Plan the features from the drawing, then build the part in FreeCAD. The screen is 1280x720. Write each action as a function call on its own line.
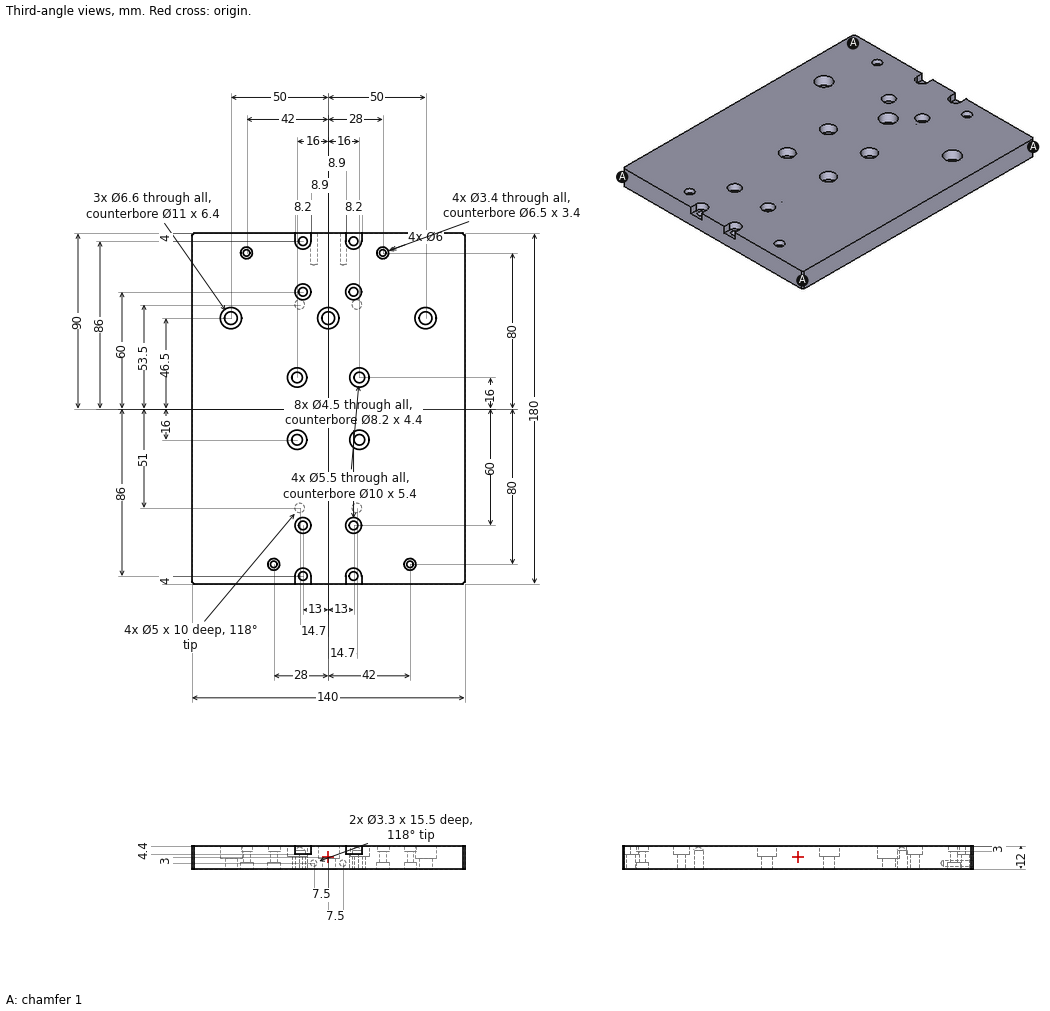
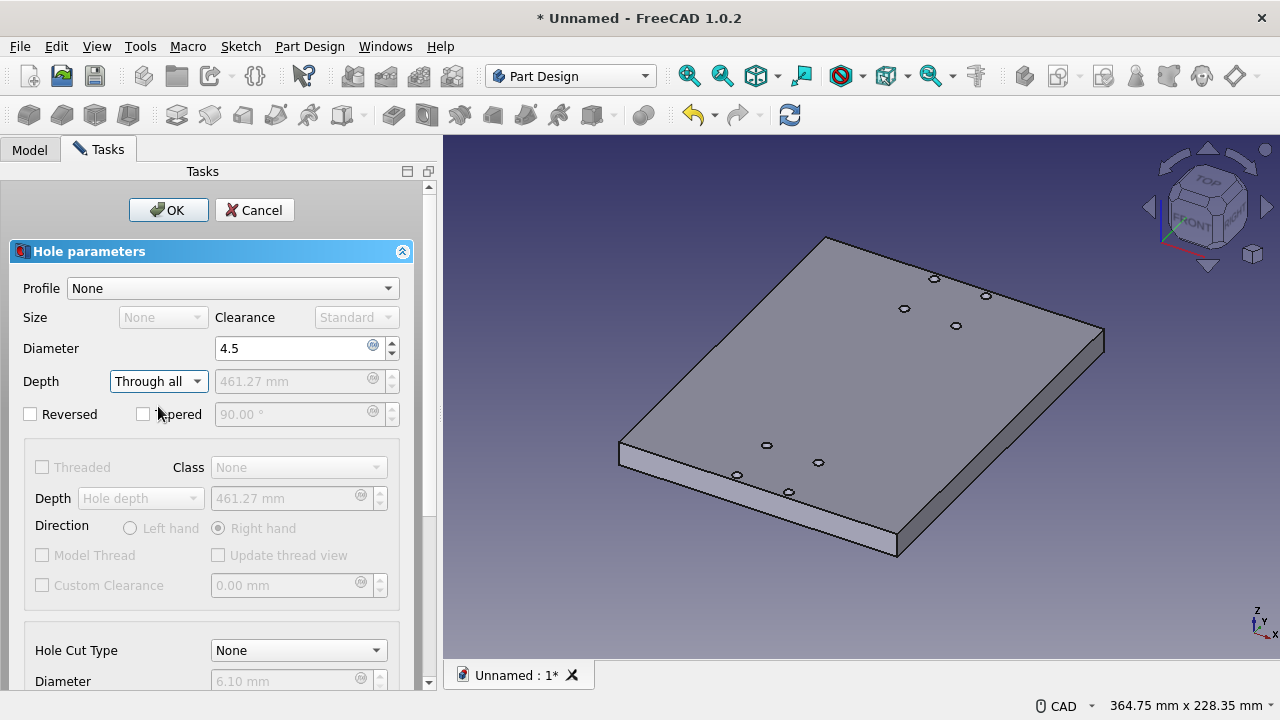
click(300, 650)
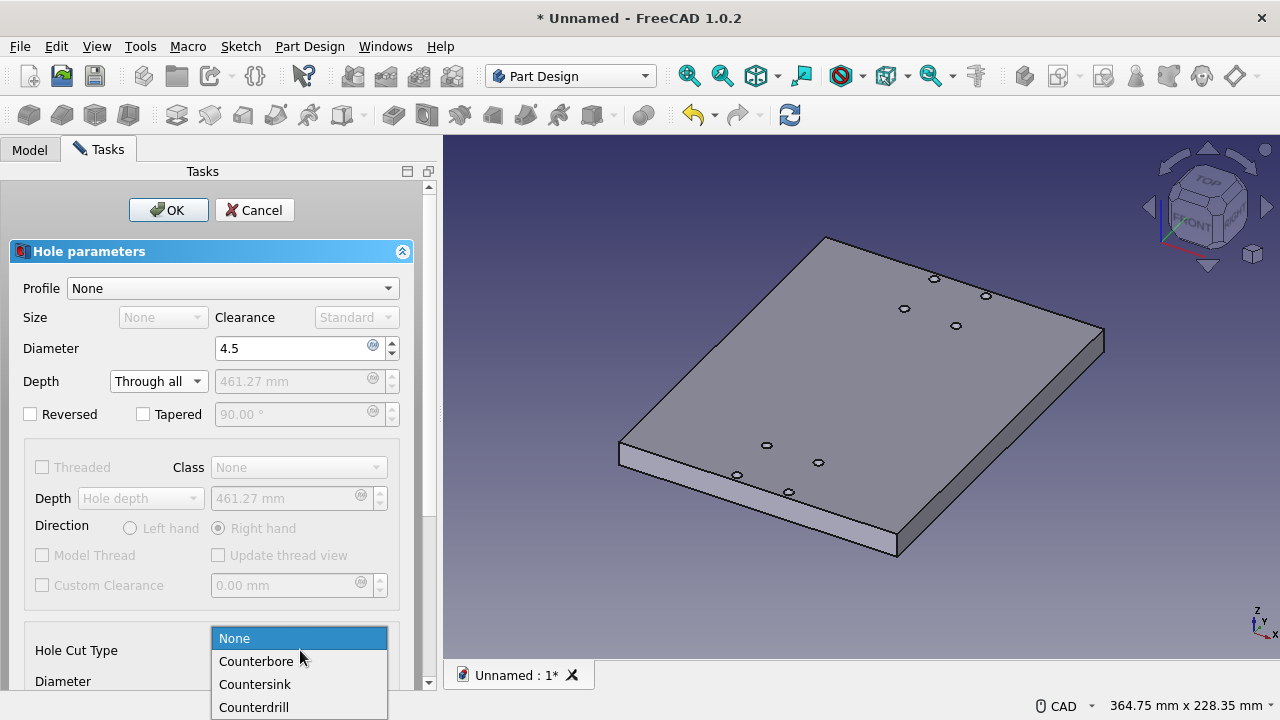
click(298, 662)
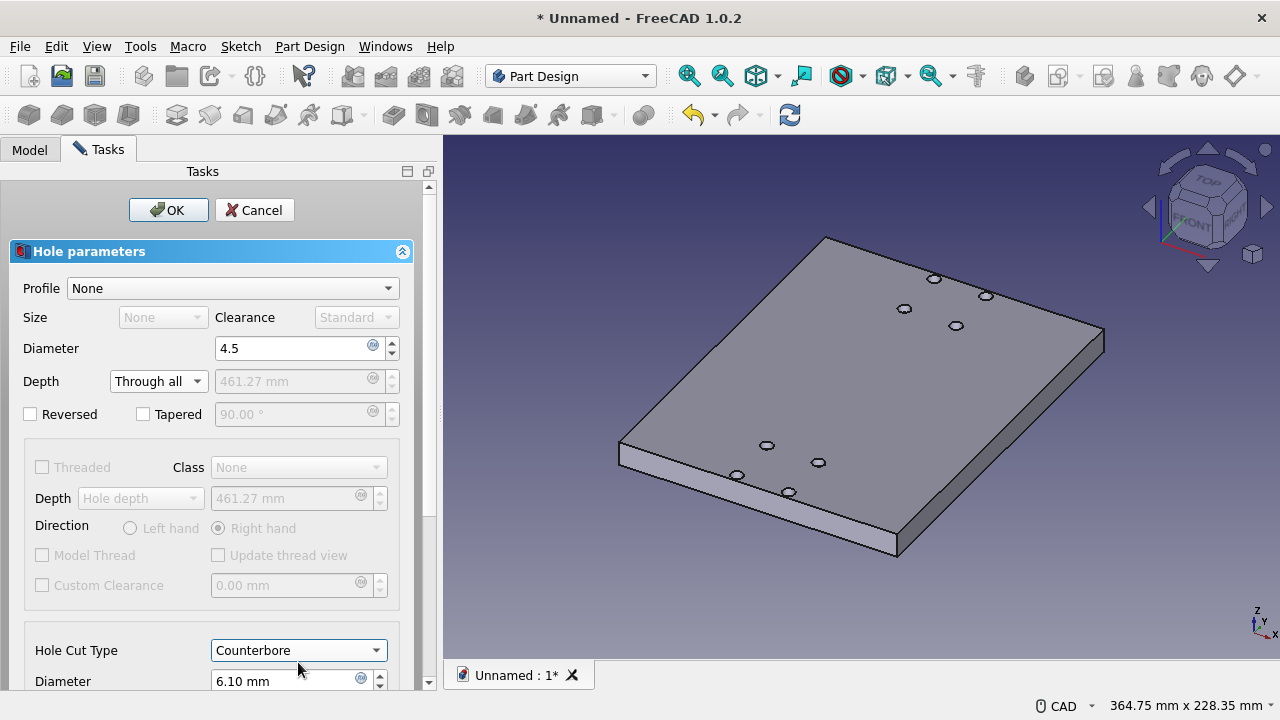
scroll(429, 436, down, 2)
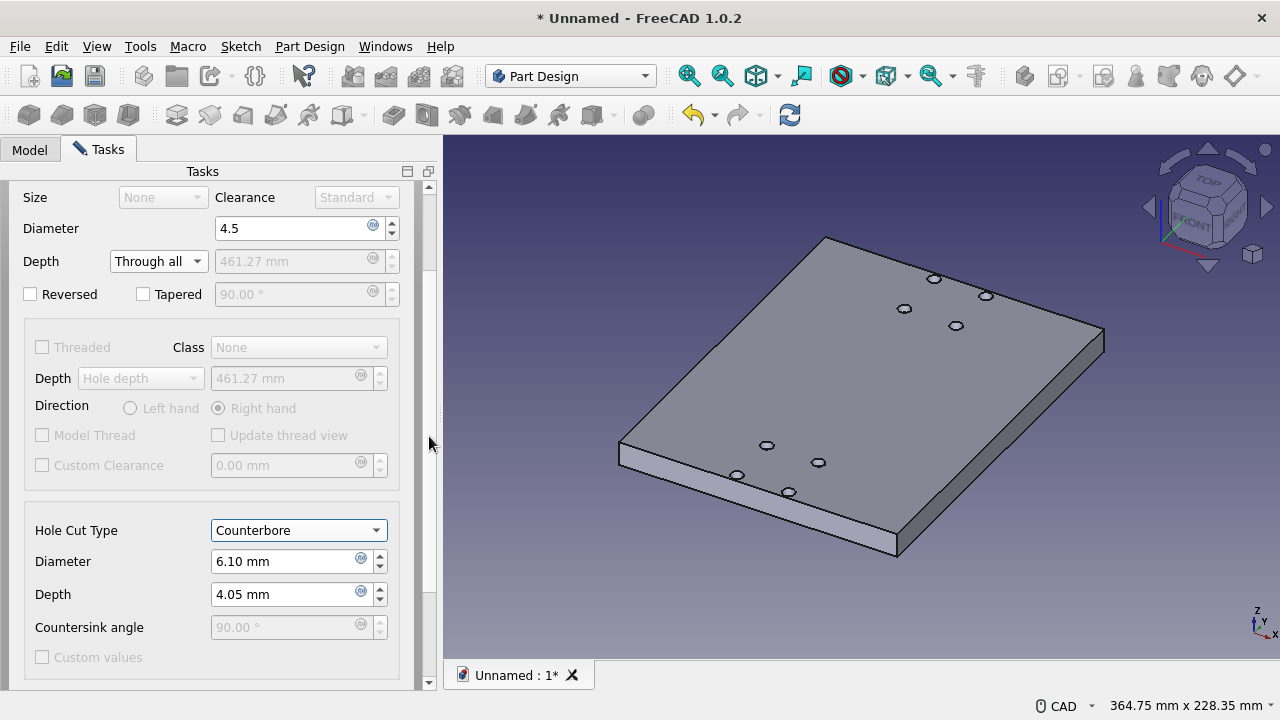
triple_click(292, 562)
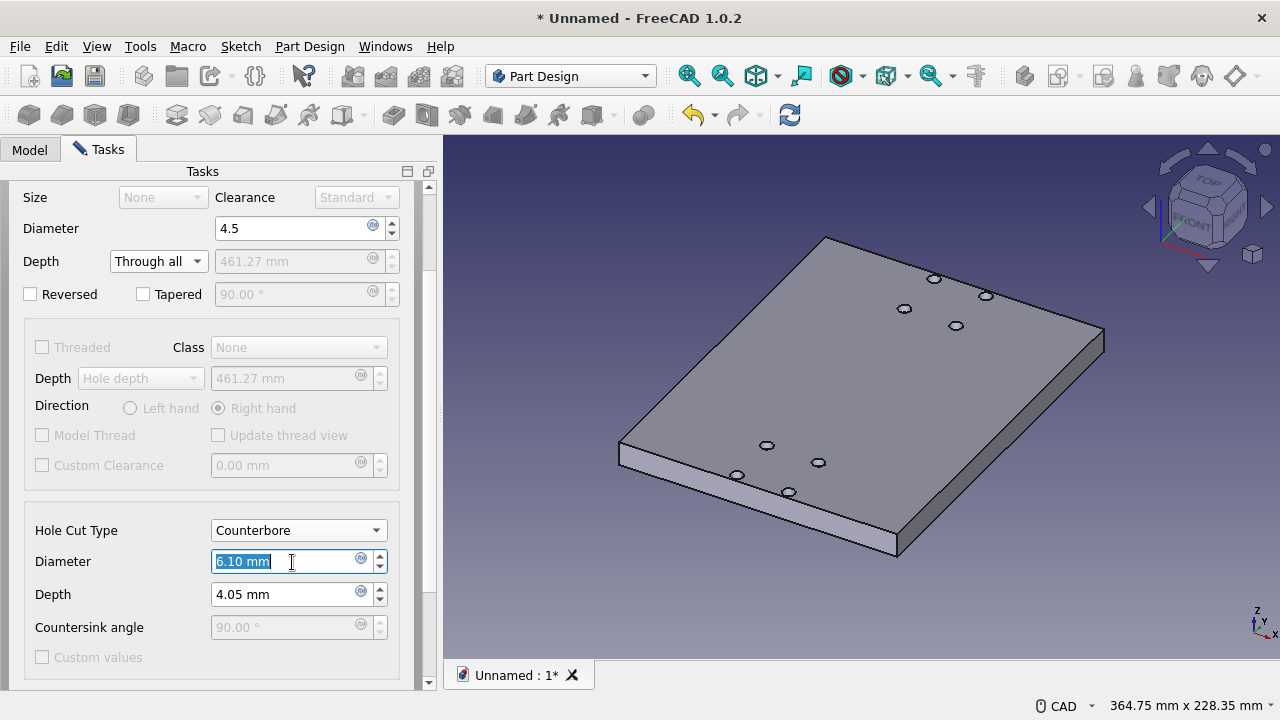
text(8.2)
key(Tab)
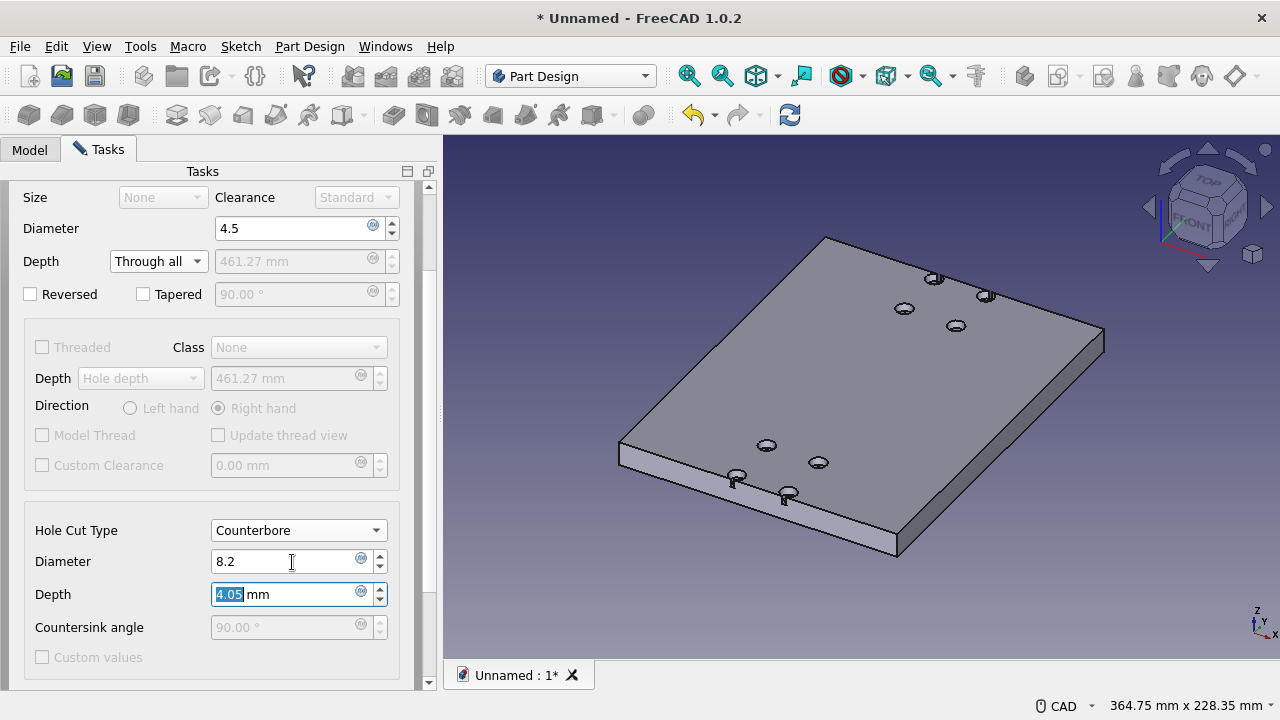
text(4.4)
key(Tab)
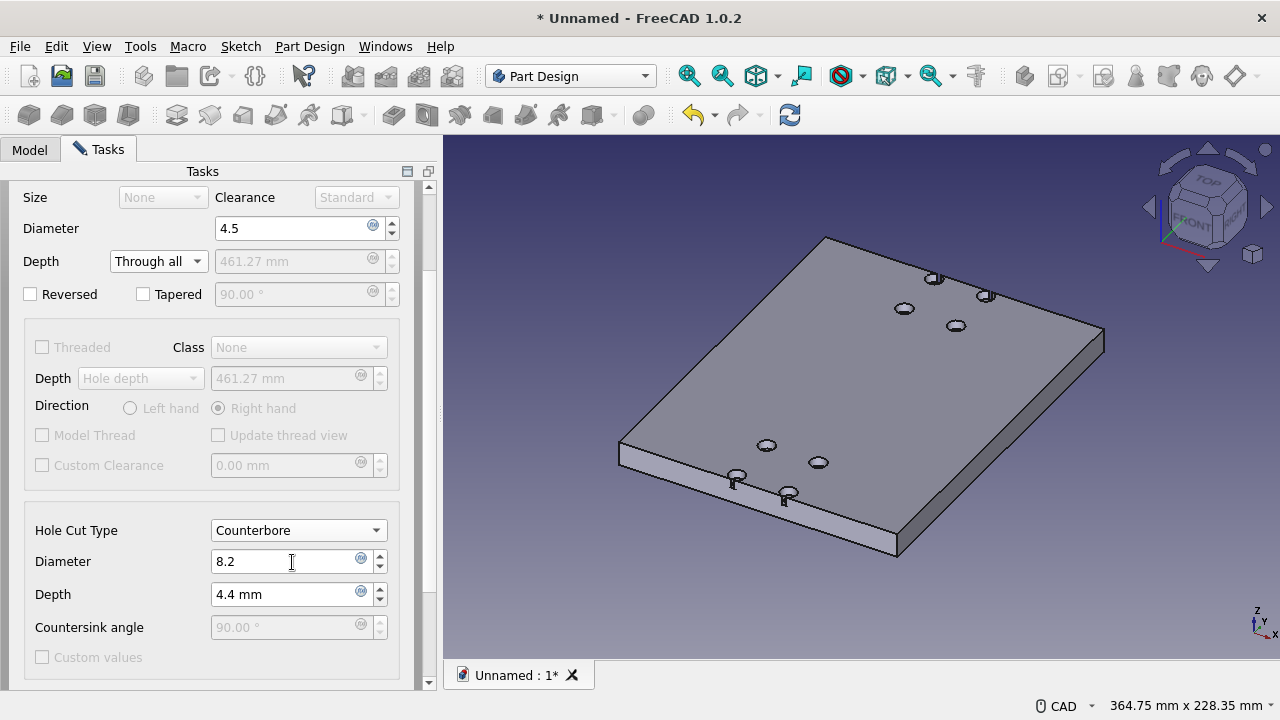
scroll(429, 436, up, 3)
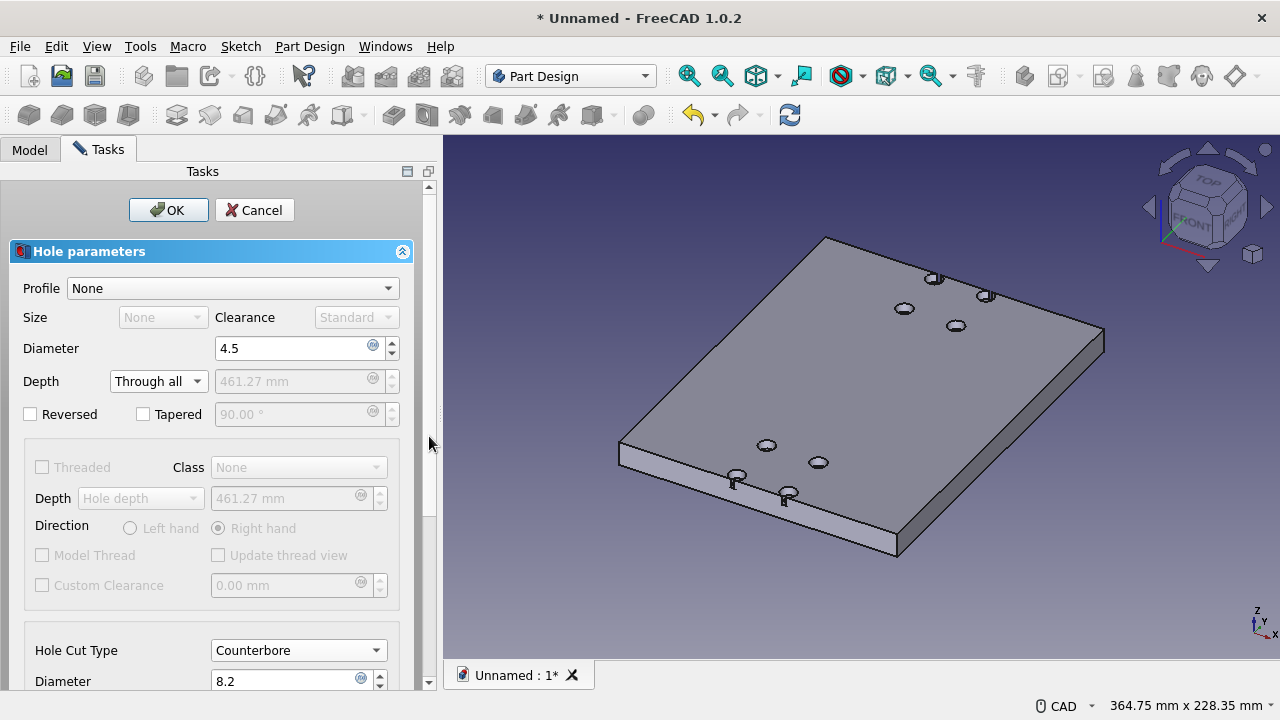
click(169, 210)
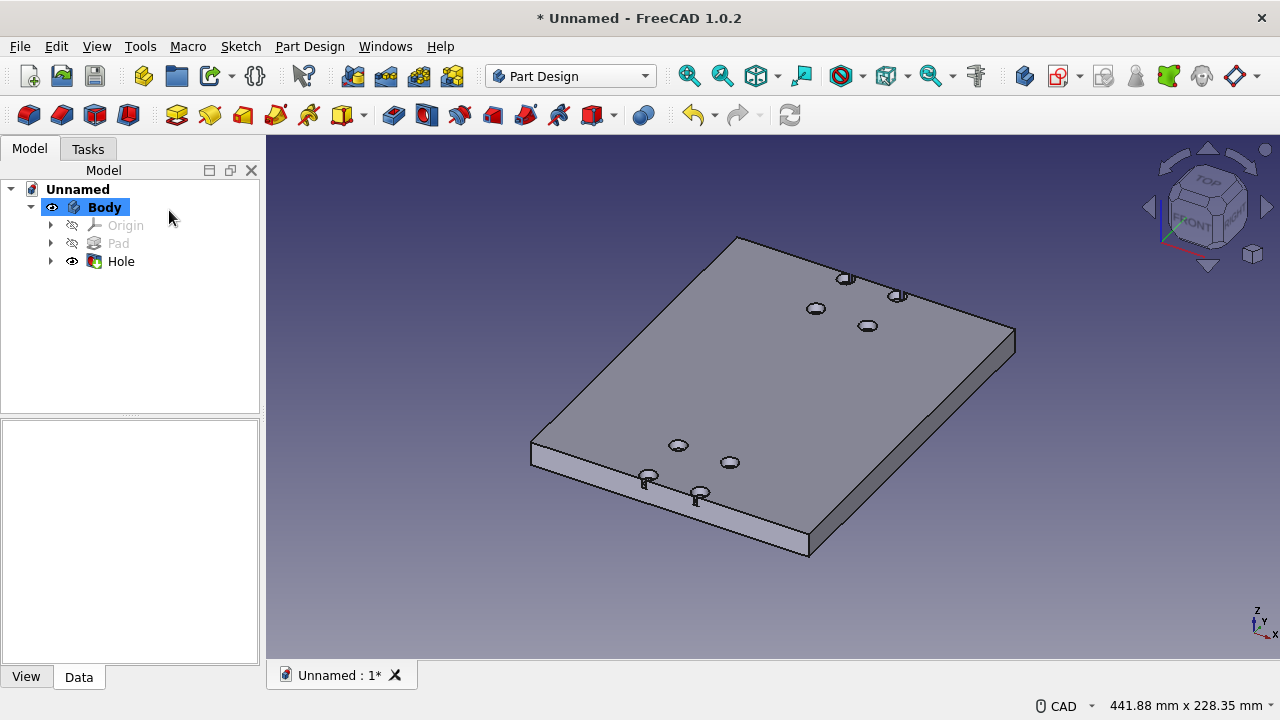
key(5)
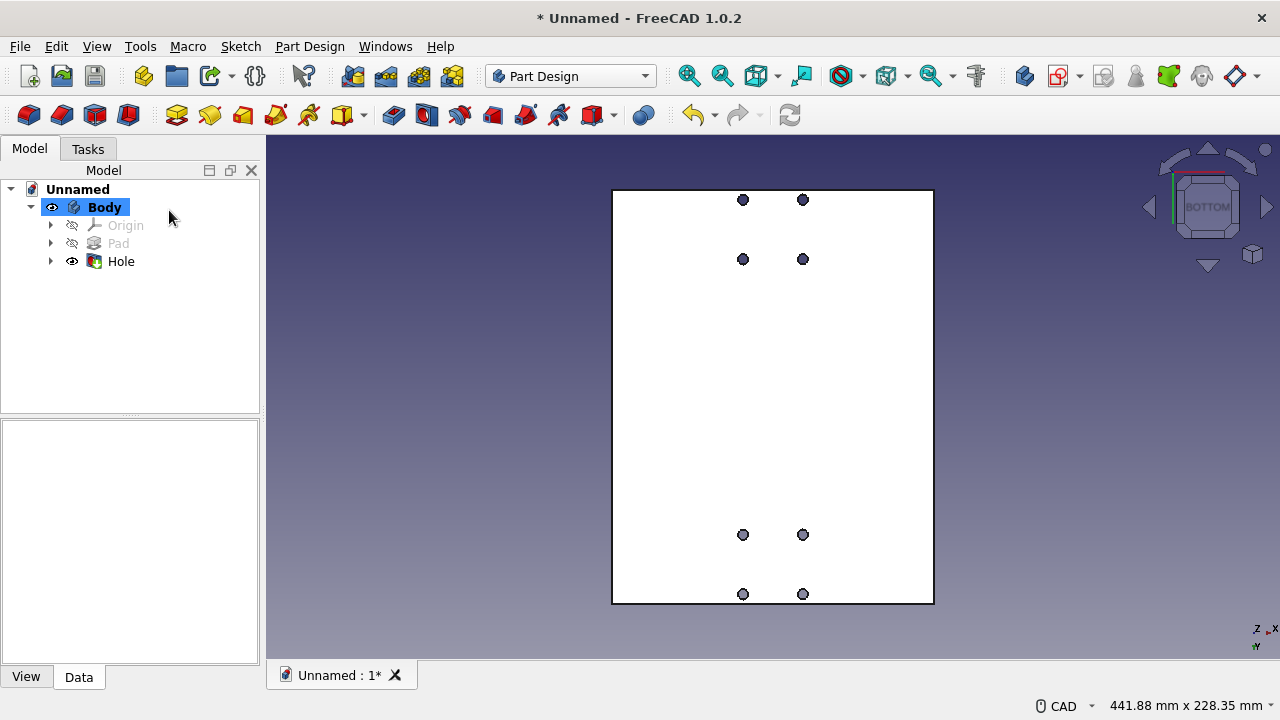
click(773, 396)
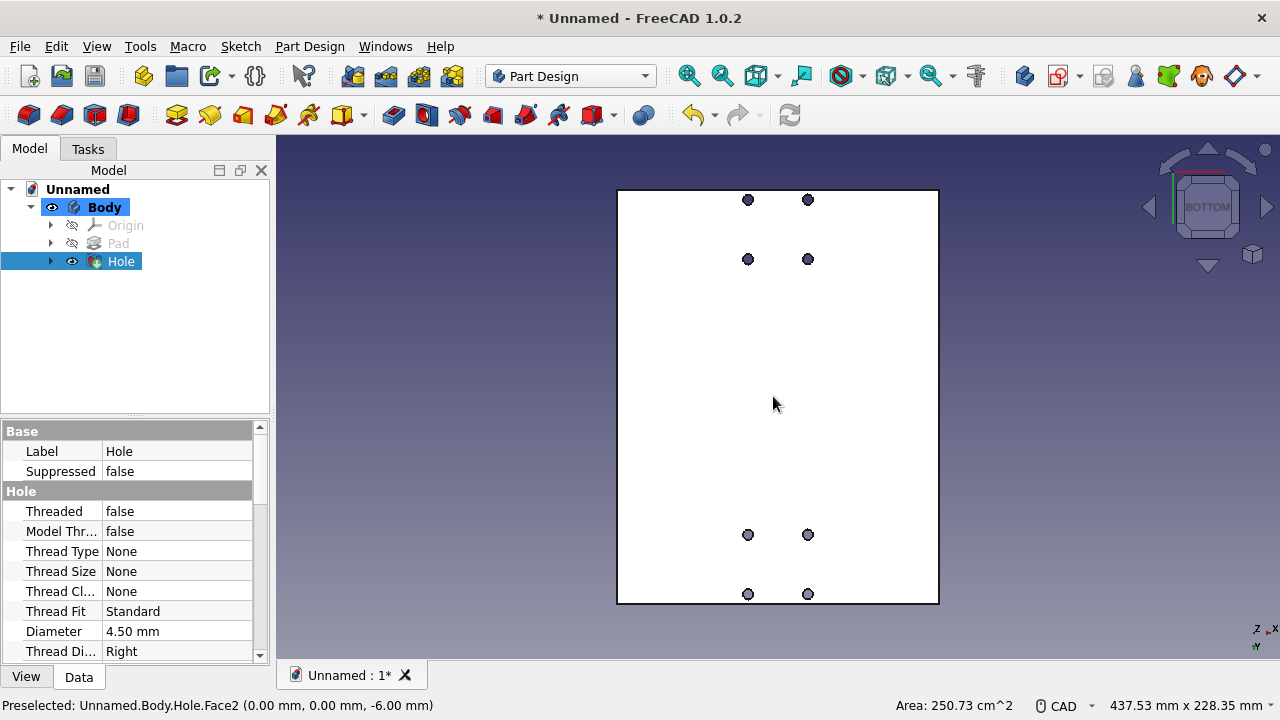
click(1058, 76)